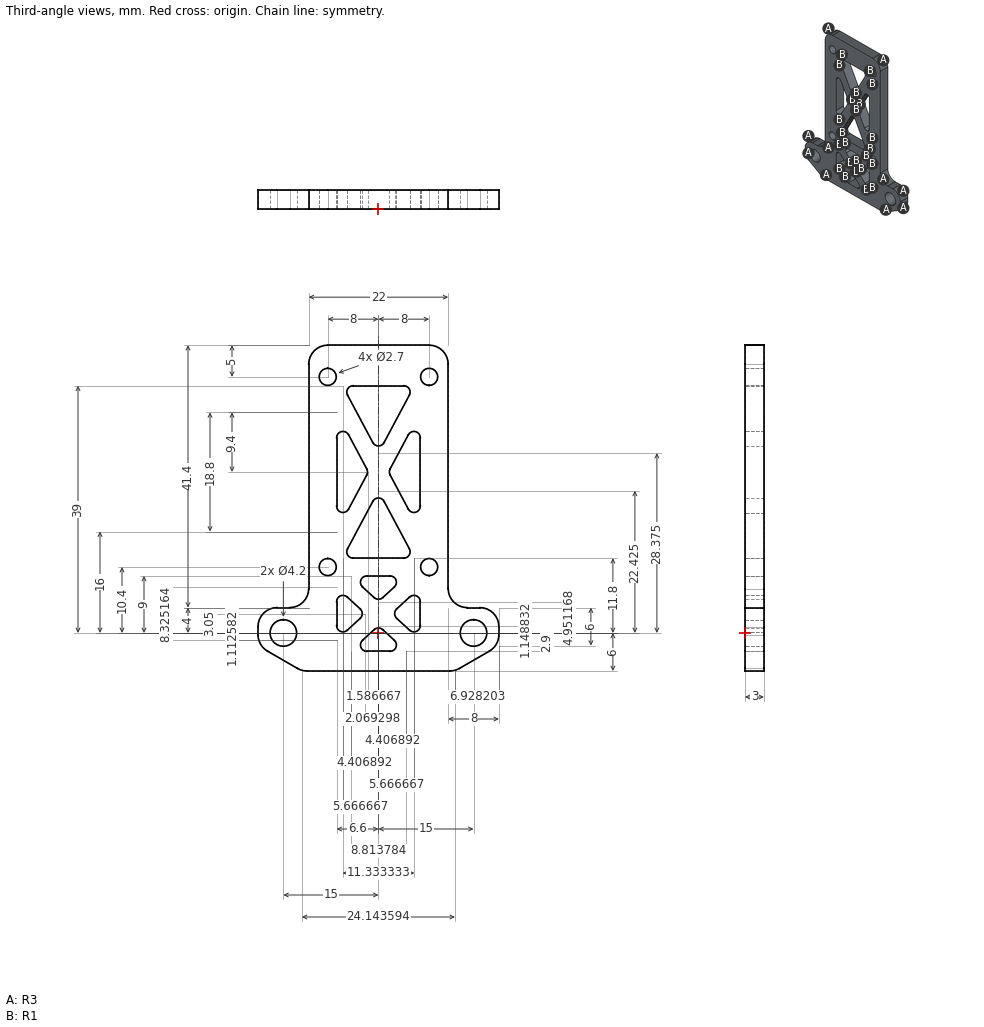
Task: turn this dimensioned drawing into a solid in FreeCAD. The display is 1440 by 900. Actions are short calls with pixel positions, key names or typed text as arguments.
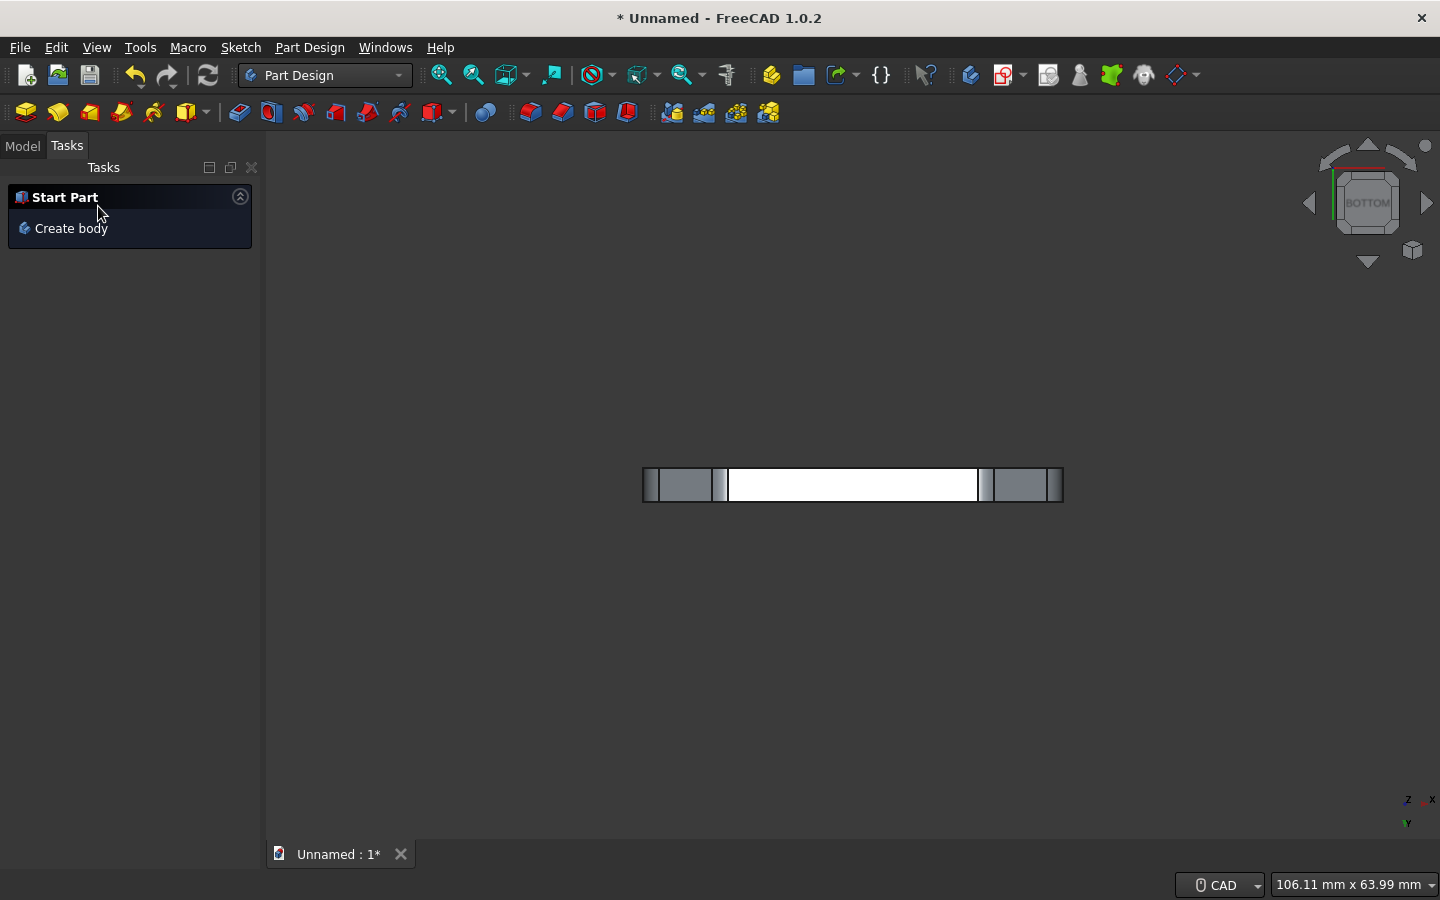
click(442, 76)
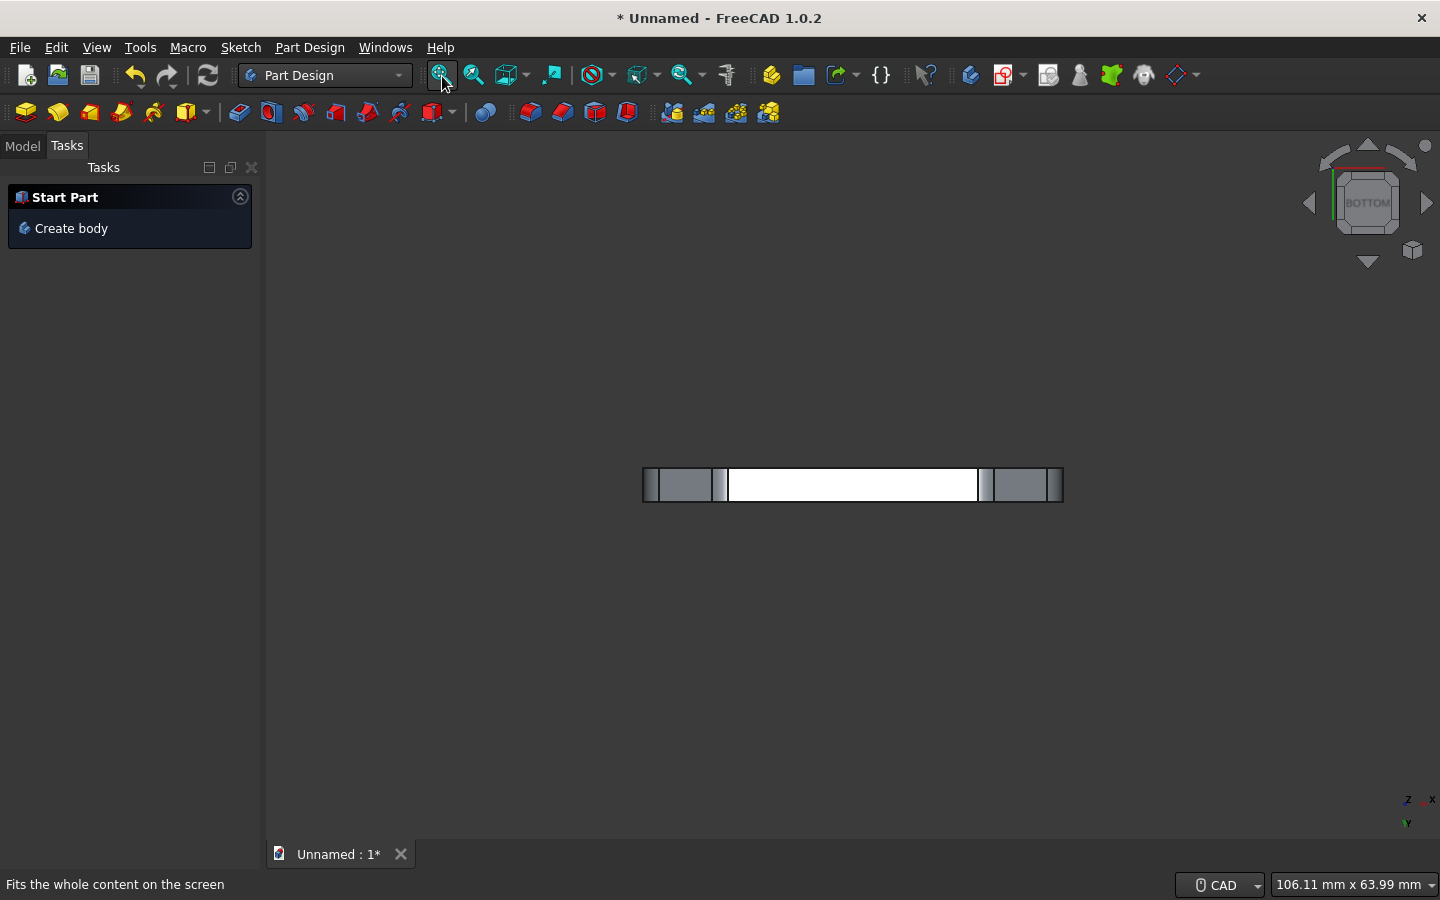
key(4)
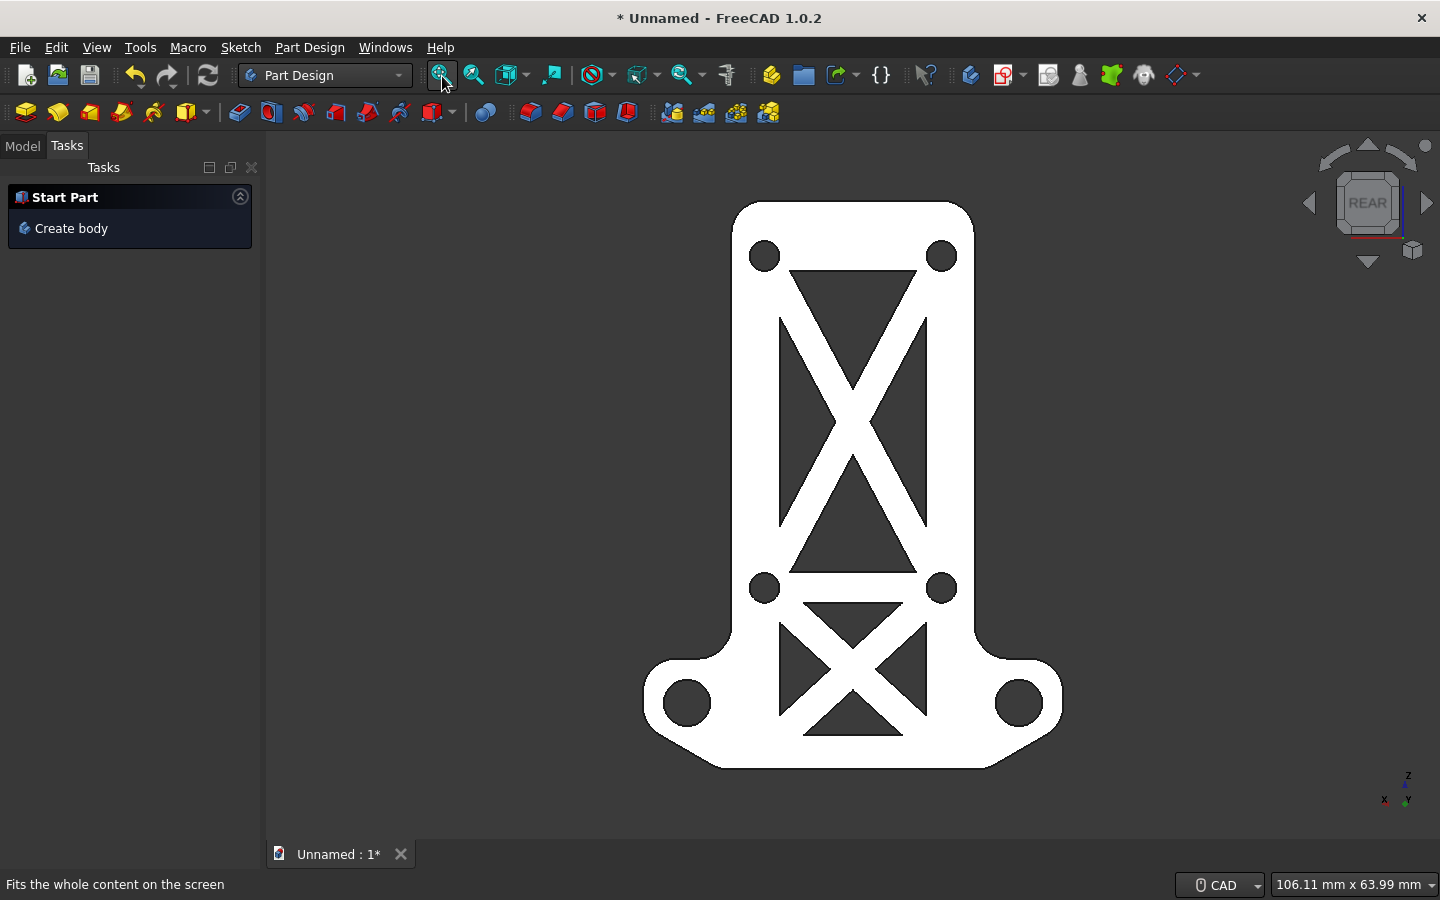
key(6)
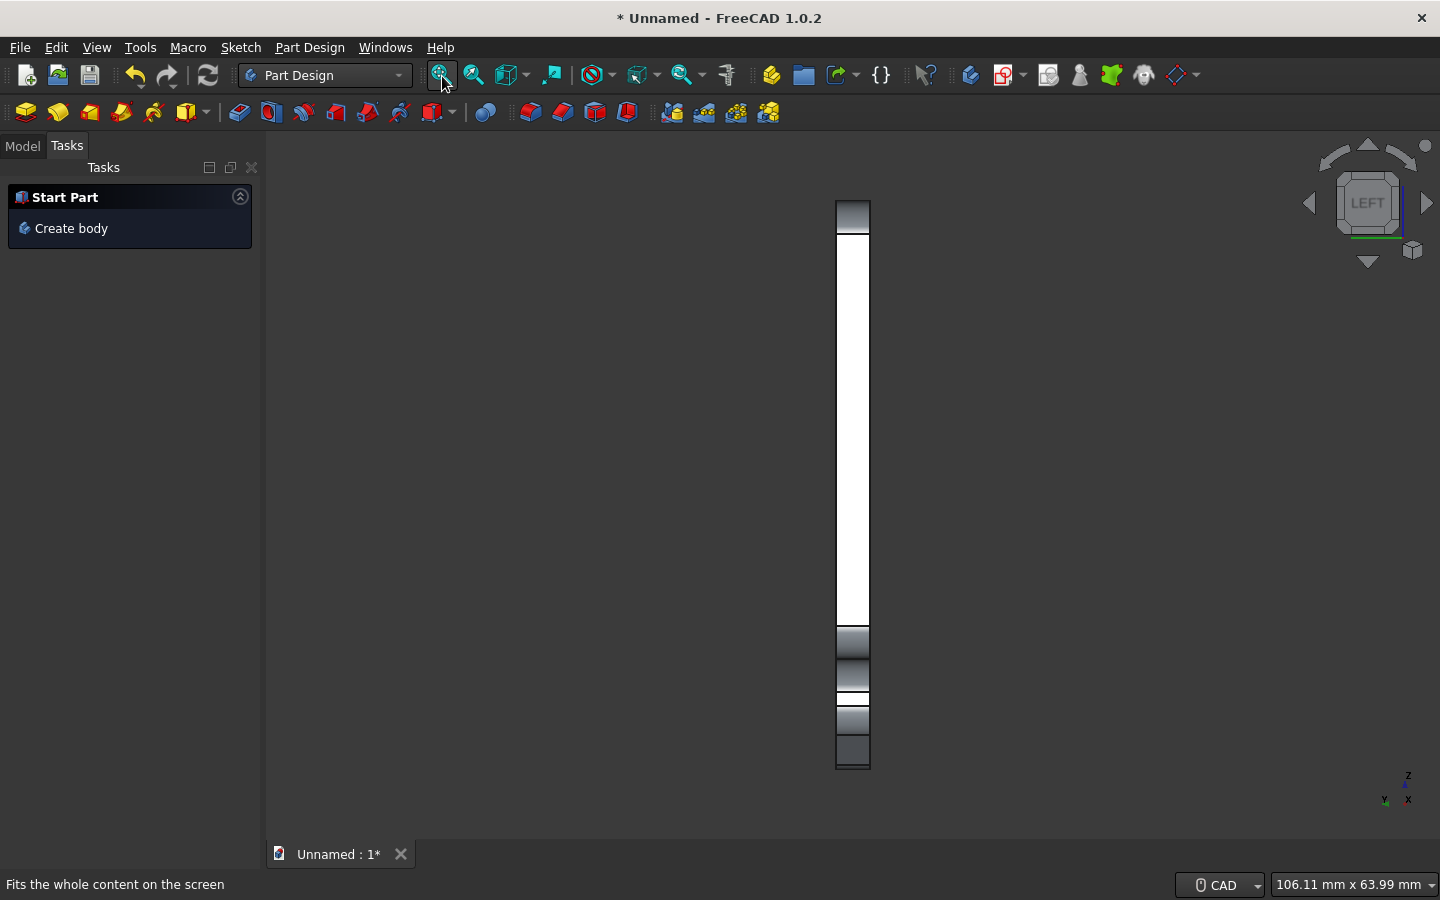
key(v)
key(3)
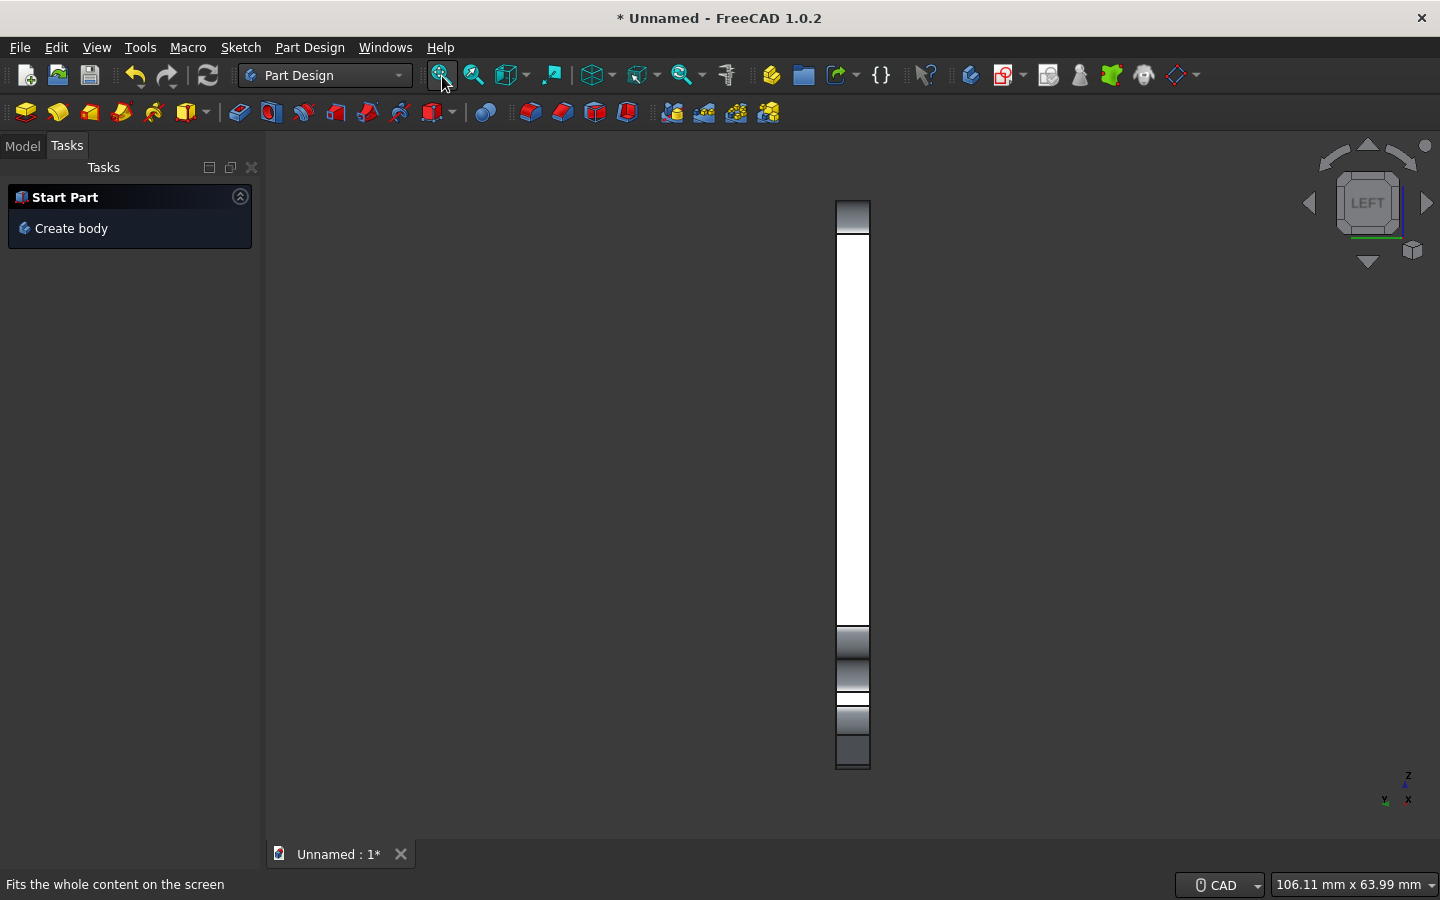
key(0)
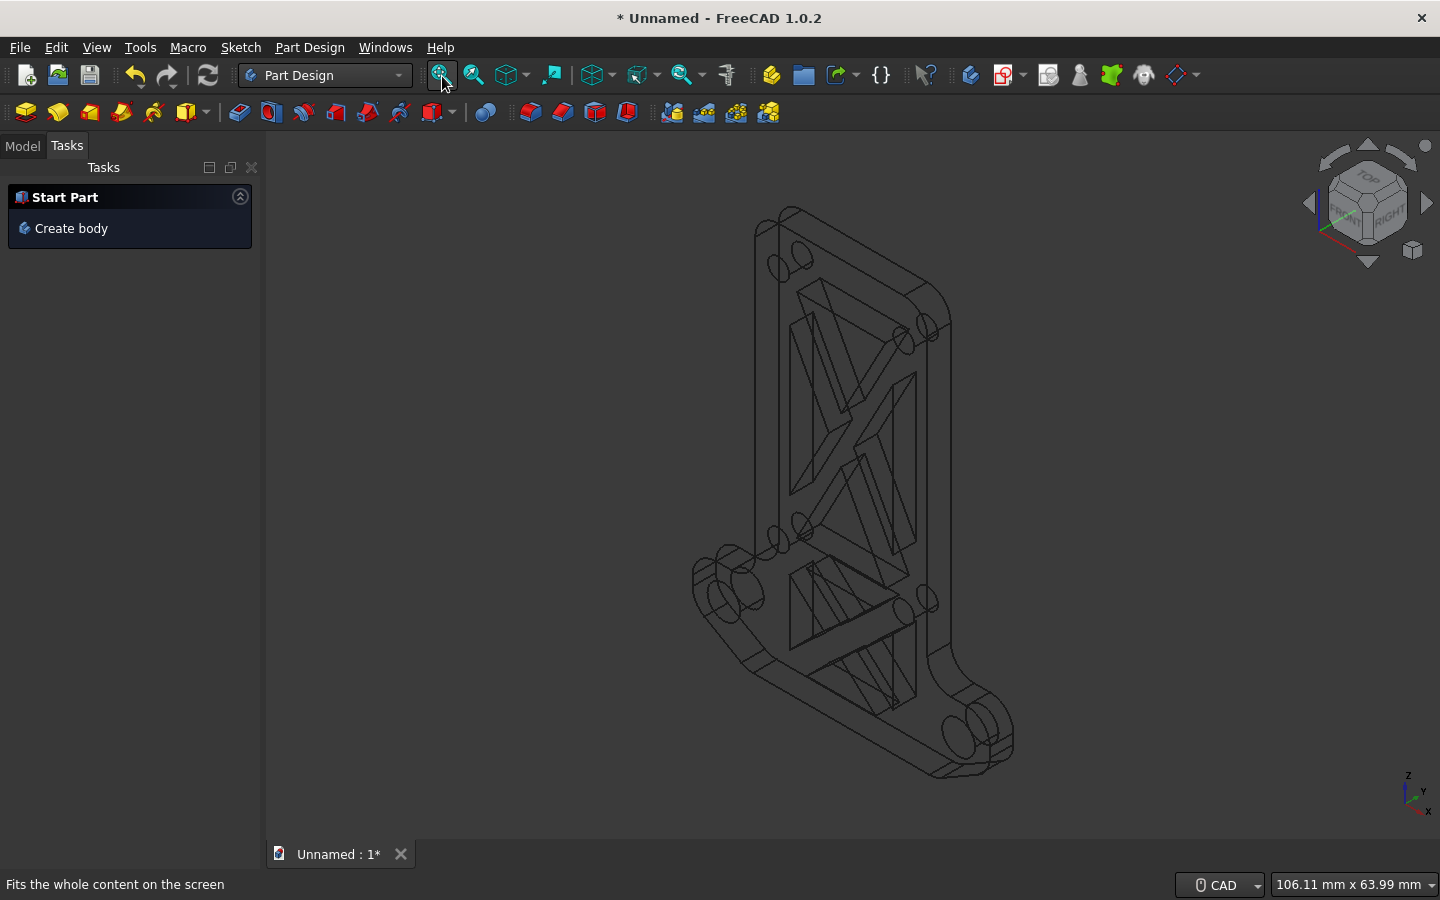
click(905, 547)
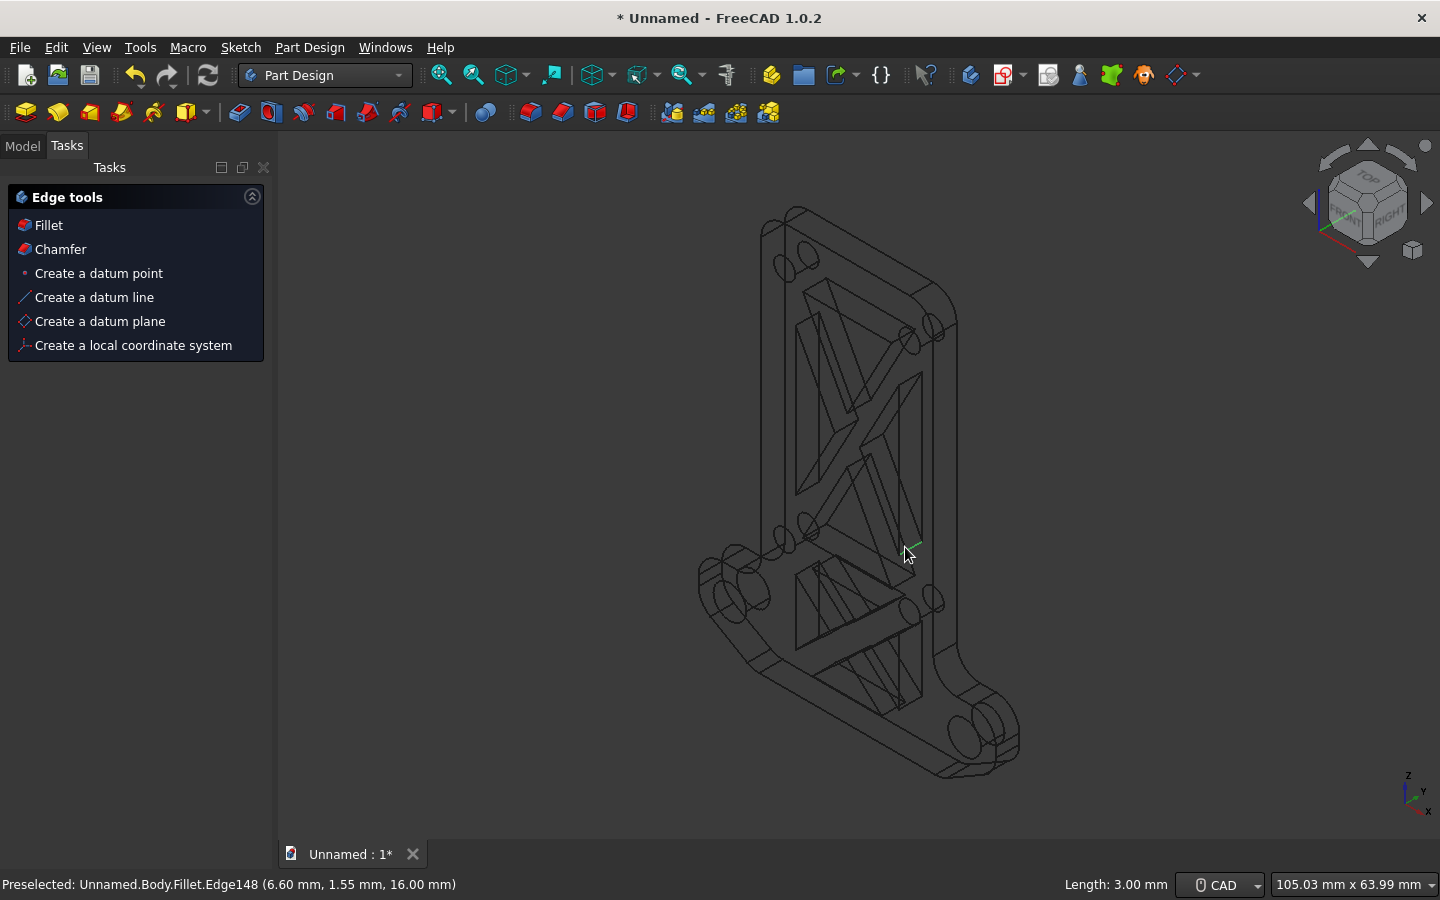
click(911, 377, ctrl)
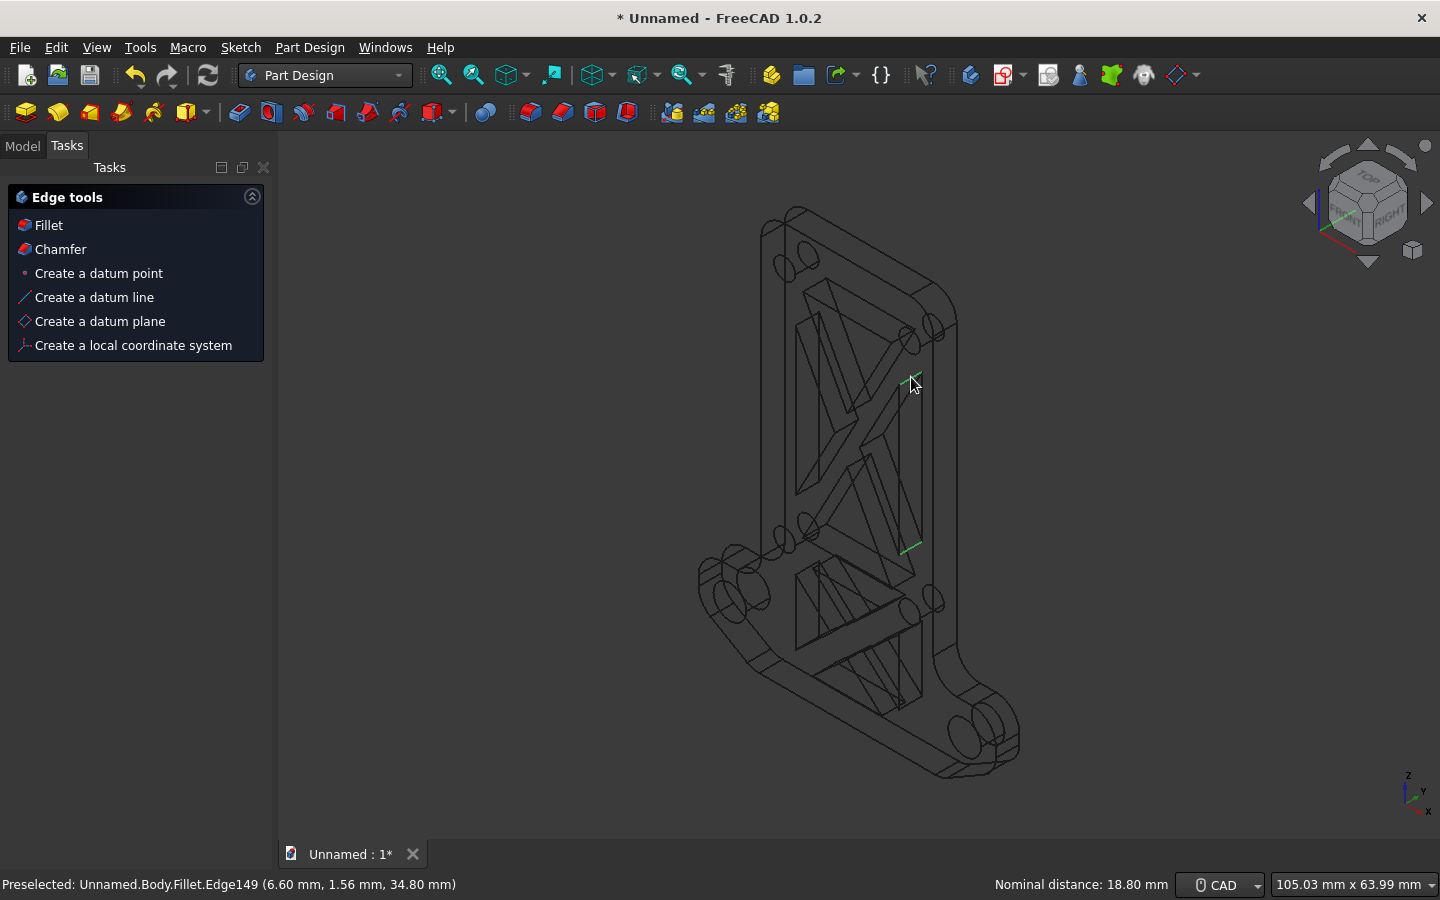
click(874, 438, ctrl)